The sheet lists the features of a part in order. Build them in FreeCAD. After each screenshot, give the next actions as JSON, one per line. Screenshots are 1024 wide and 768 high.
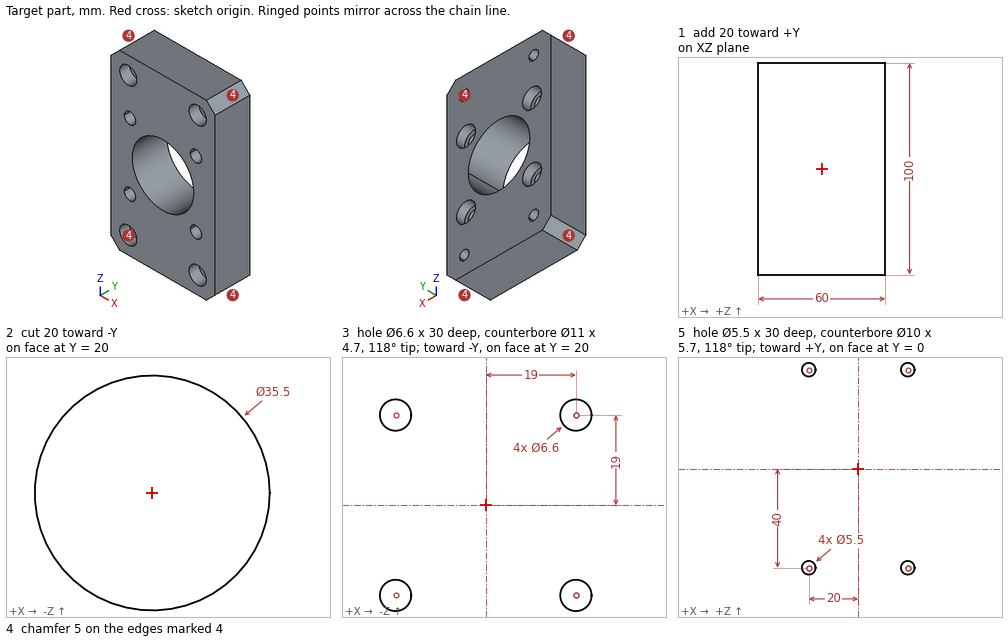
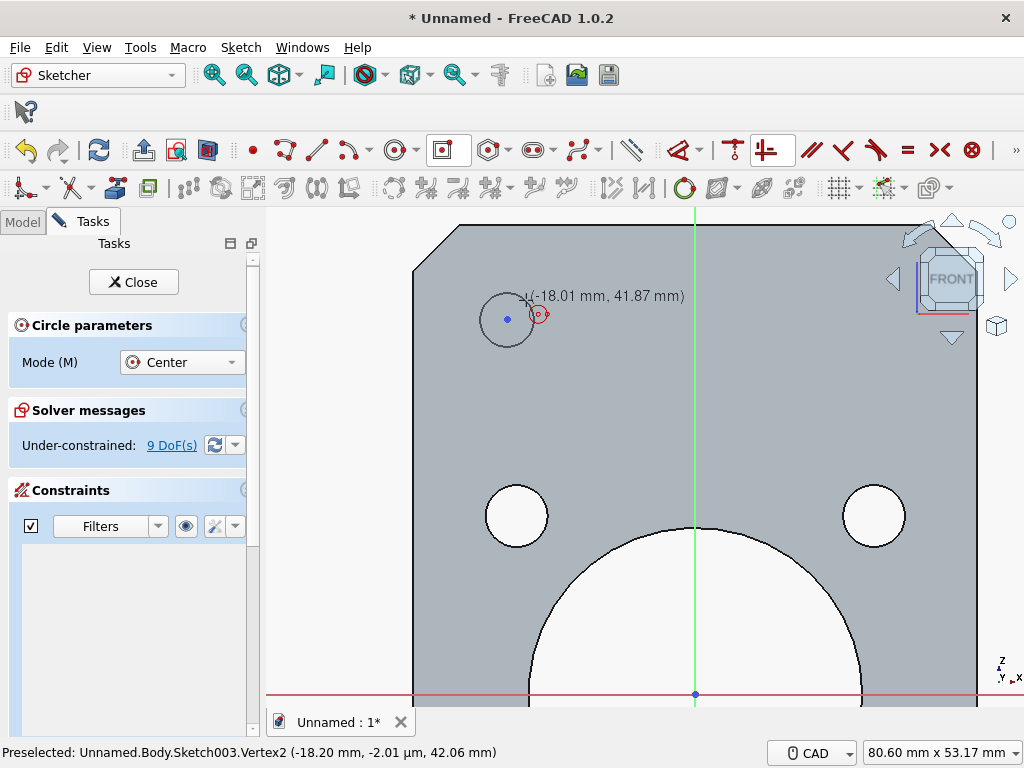
{"action": "scroll", "coordinate": [507, 319], "scroll_direction": "down", "scroll_amount": 5}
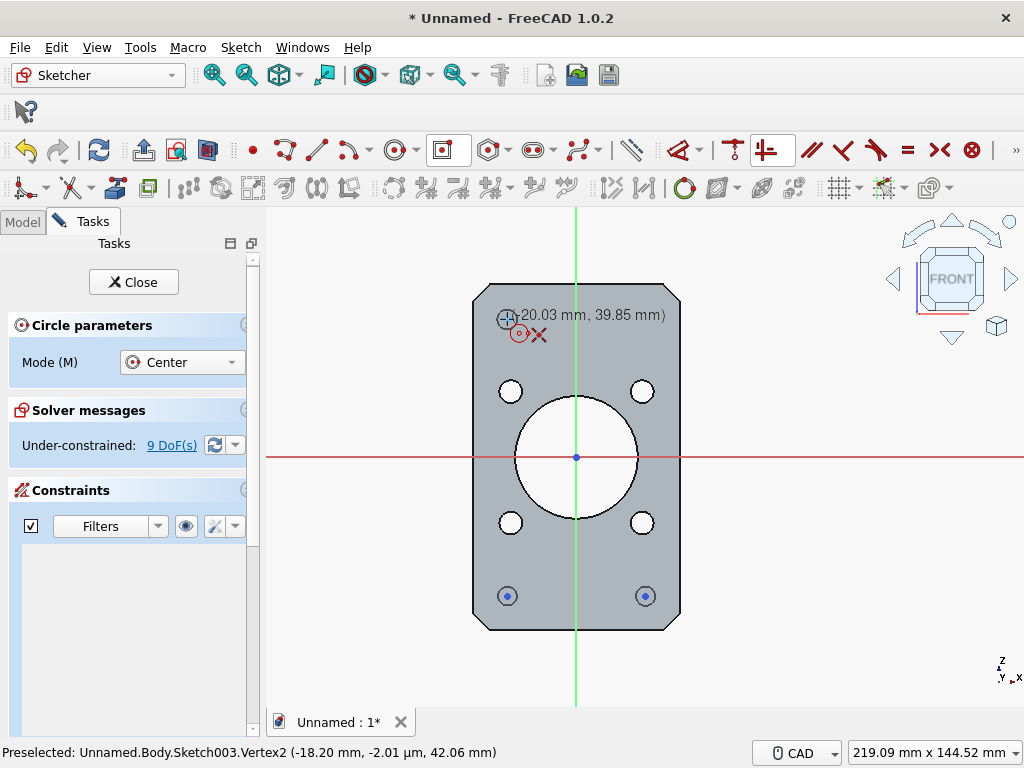
{"action": "scroll", "coordinate": [646, 319], "scroll_direction": "up", "scroll_amount": 5}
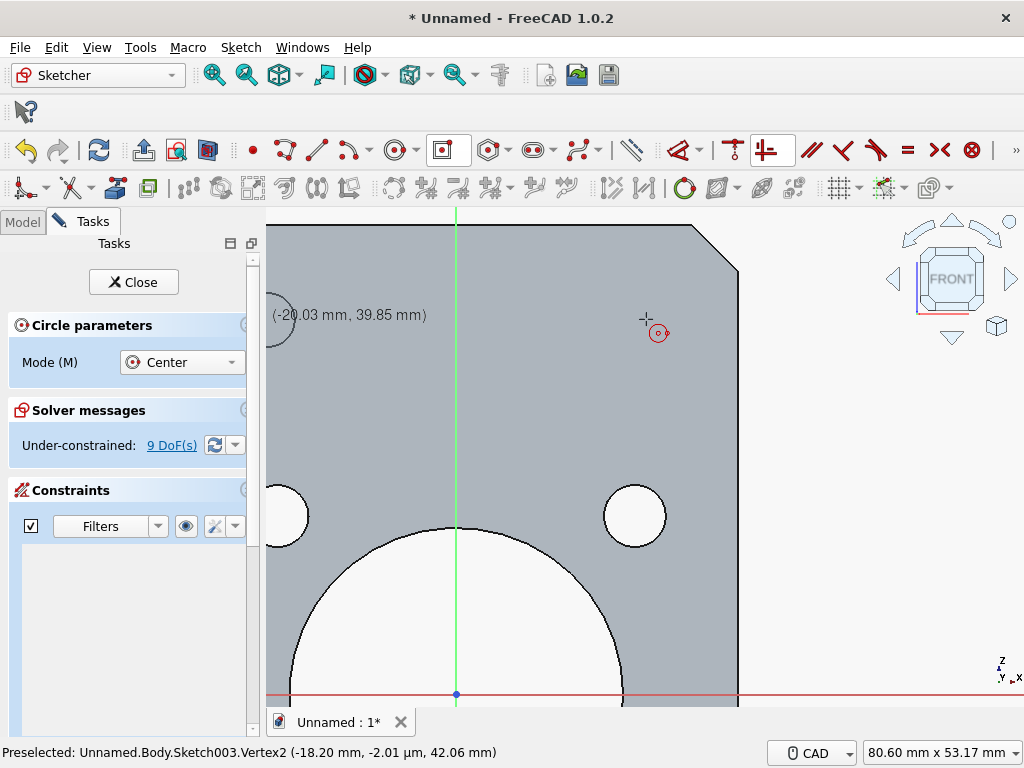
{"action": "left_click", "coordinate": [644, 319]}
{"action": "left_click", "coordinate": [663, 300]}
{"action": "key", "text": "Escape"}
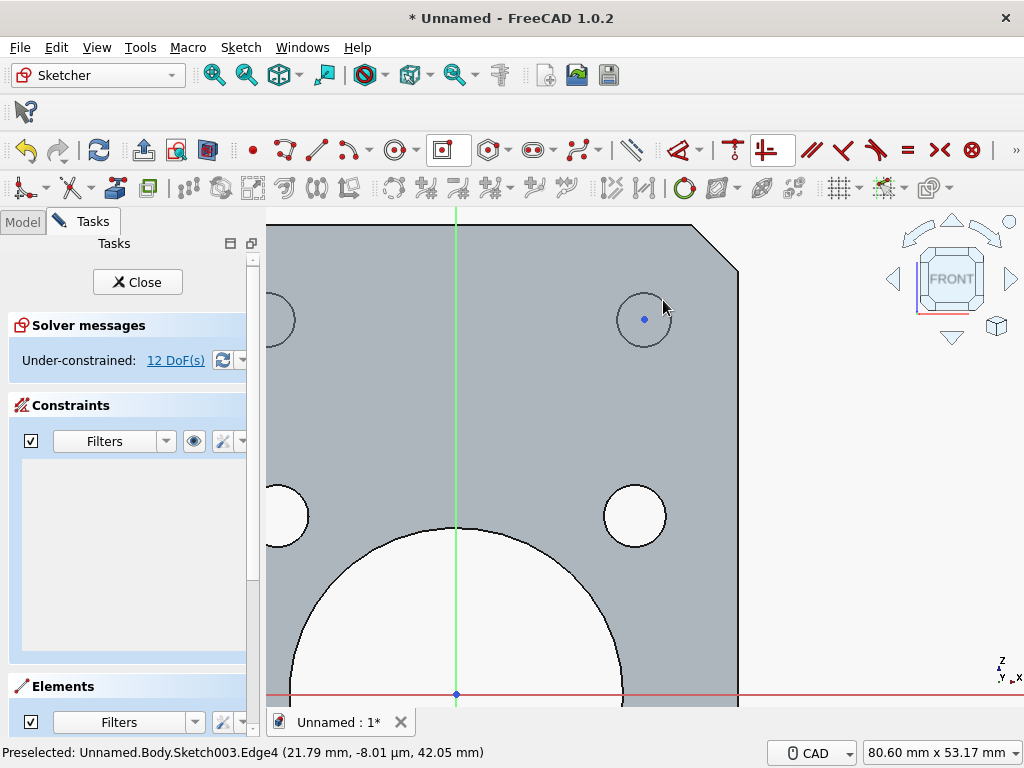
{"action": "scroll", "coordinate": [647, 319], "scroll_direction": "down", "scroll_amount": 5}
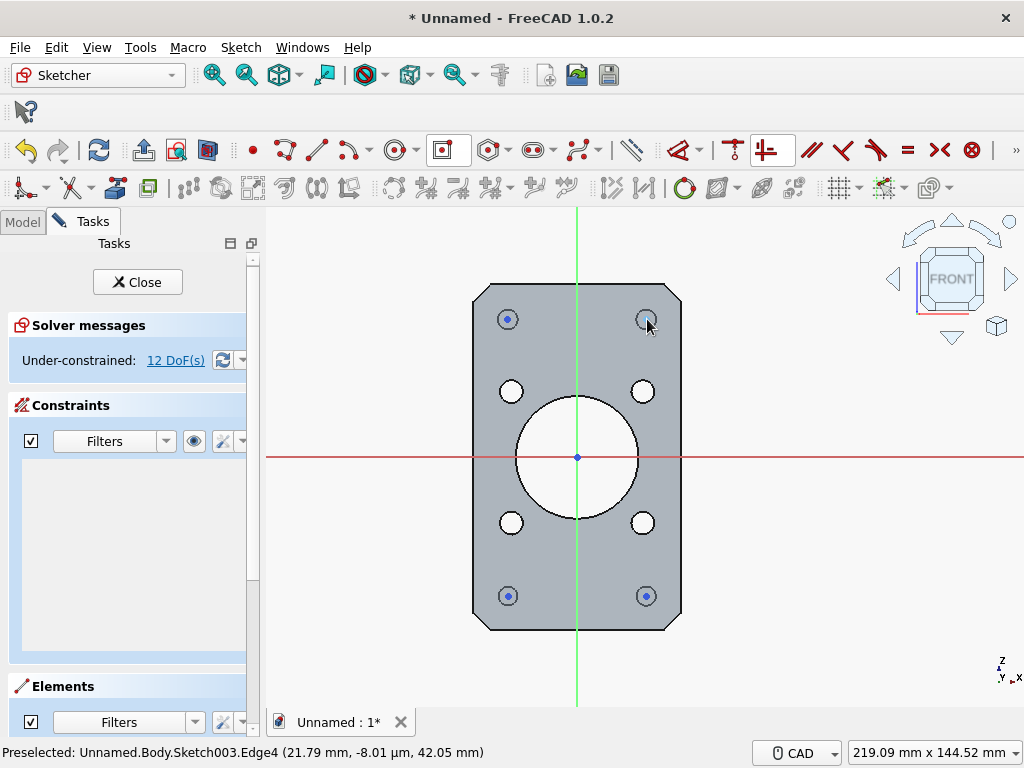
{"action": "scroll", "coordinate": [515, 589], "scroll_direction": "up", "scroll_amount": 2}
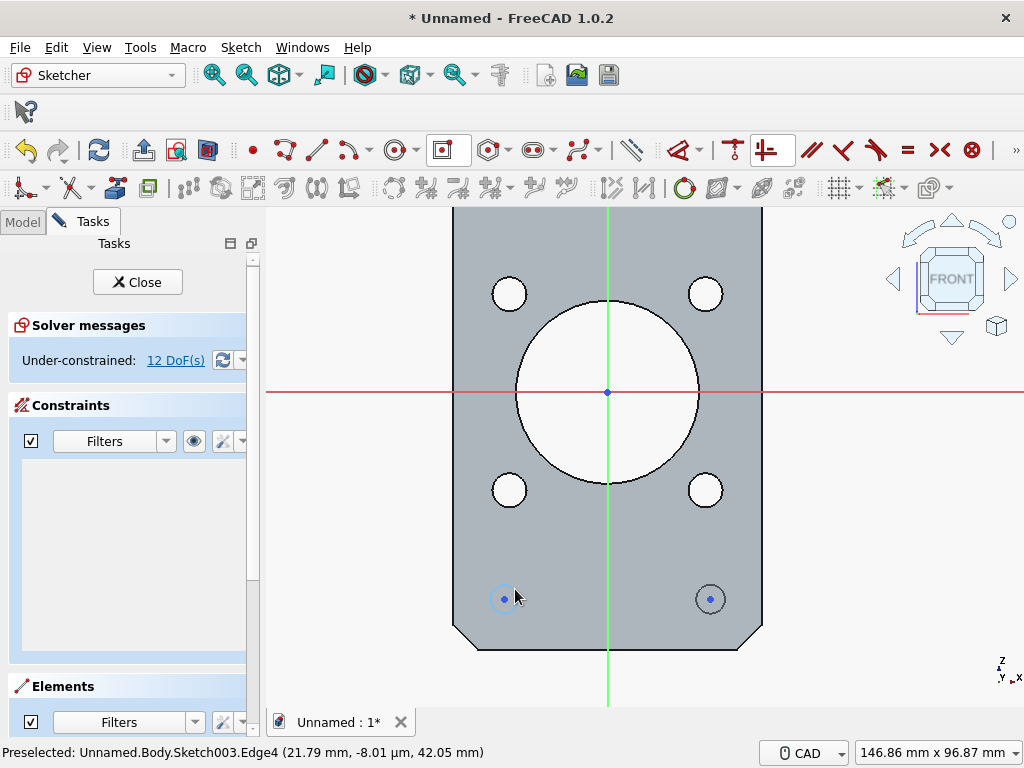
{"action": "left_click", "coordinate": [514, 589]}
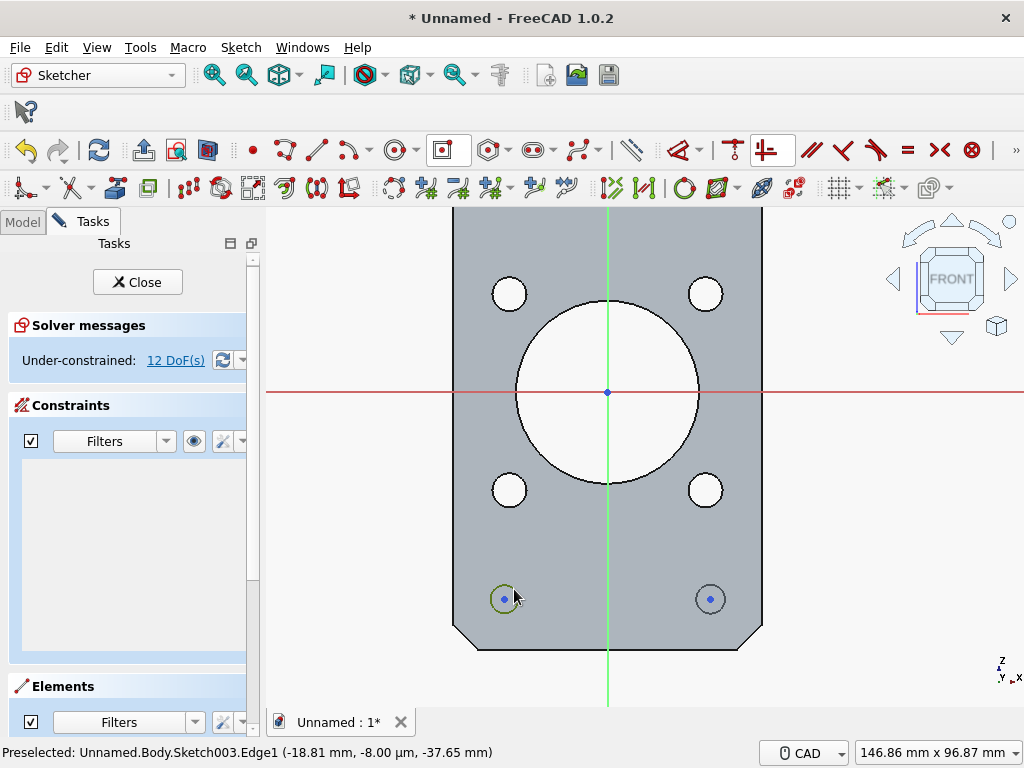
{"action": "left_click", "coordinate": [721, 589]}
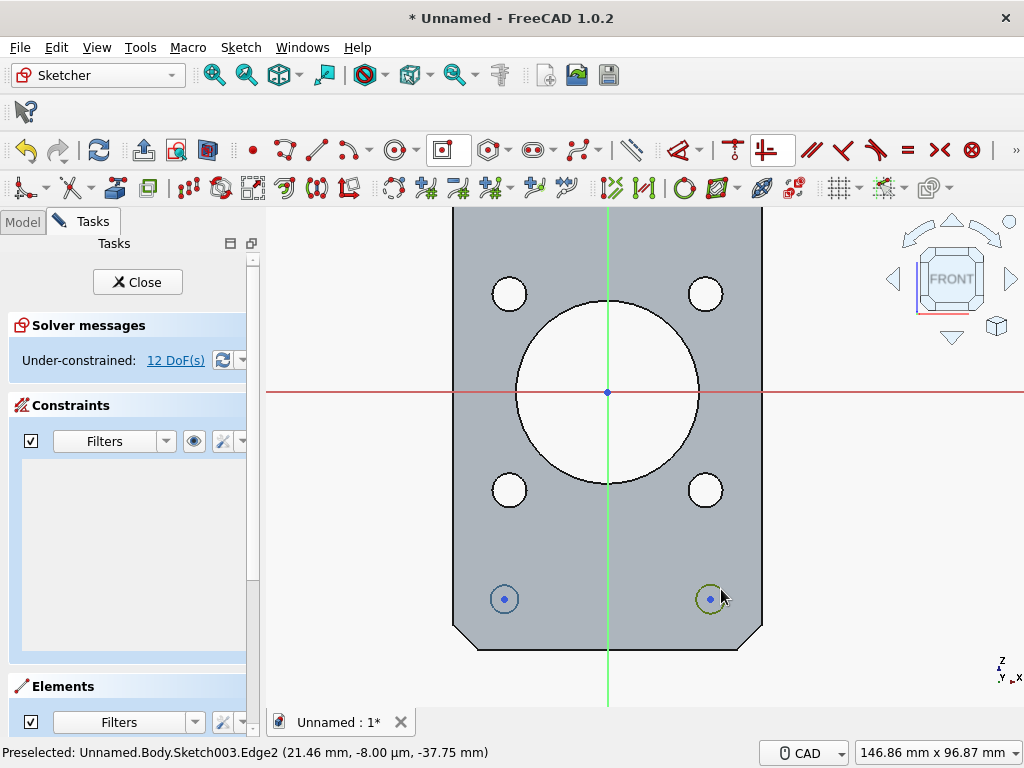
{"action": "scroll", "coordinate": [513, 589], "scroll_direction": "down", "scroll_amount": 2}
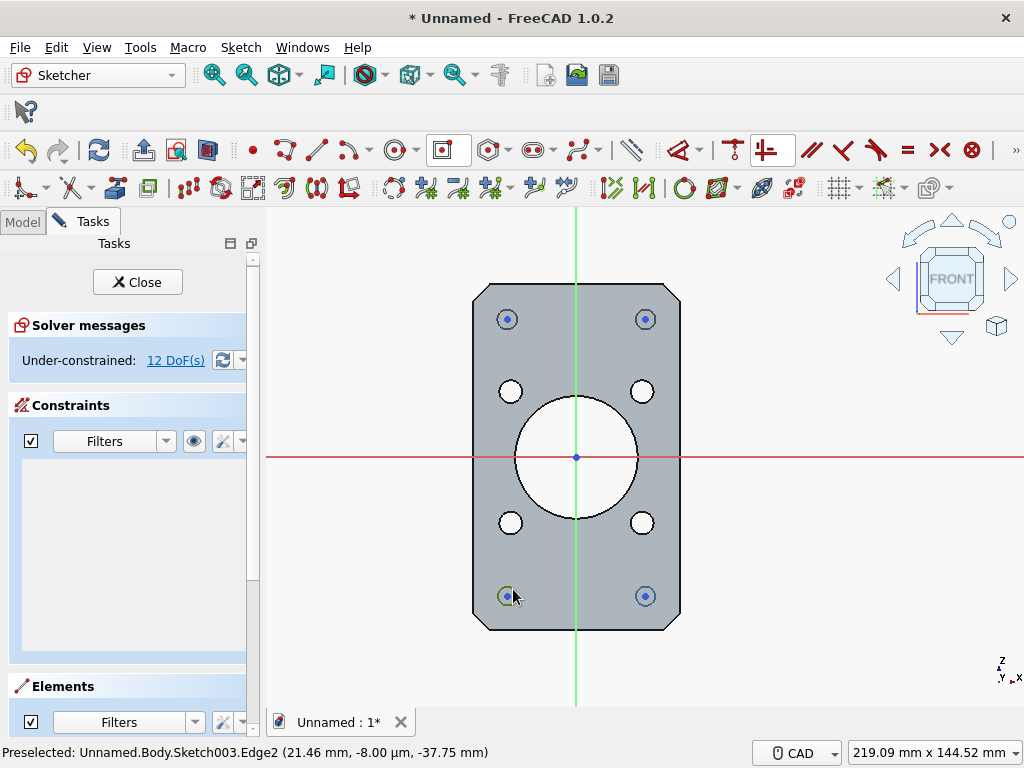
{"action": "scroll", "coordinate": [514, 312], "scroll_direction": "up", "scroll_amount": 2}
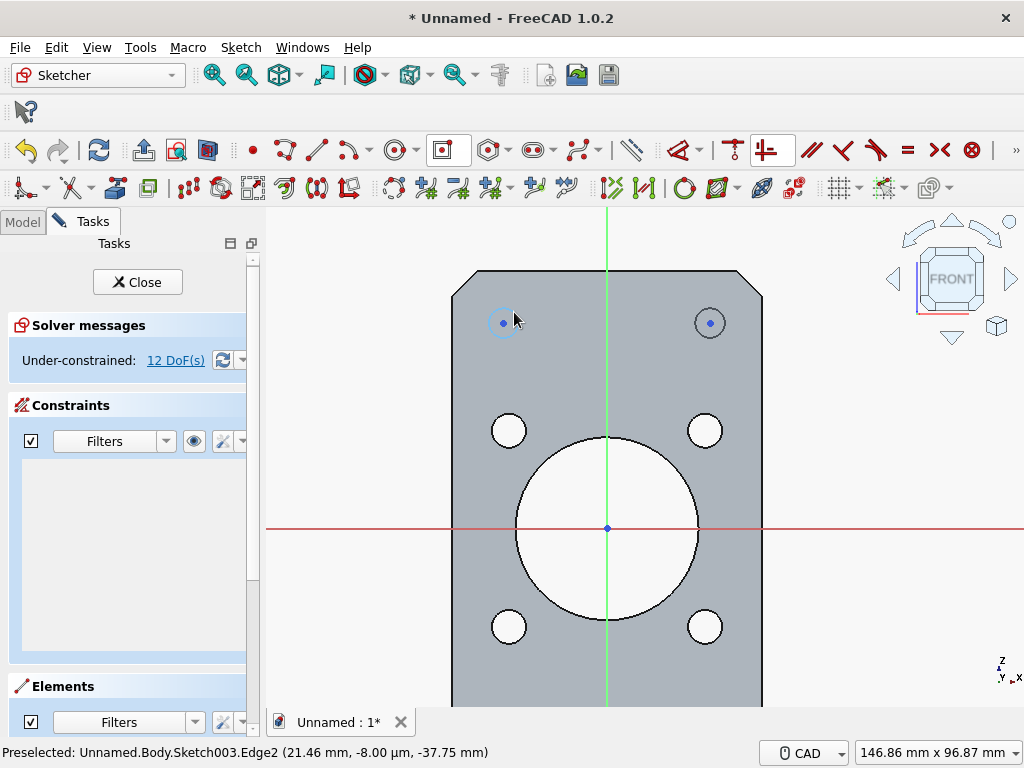
{"action": "left_click", "coordinate": [514, 313]}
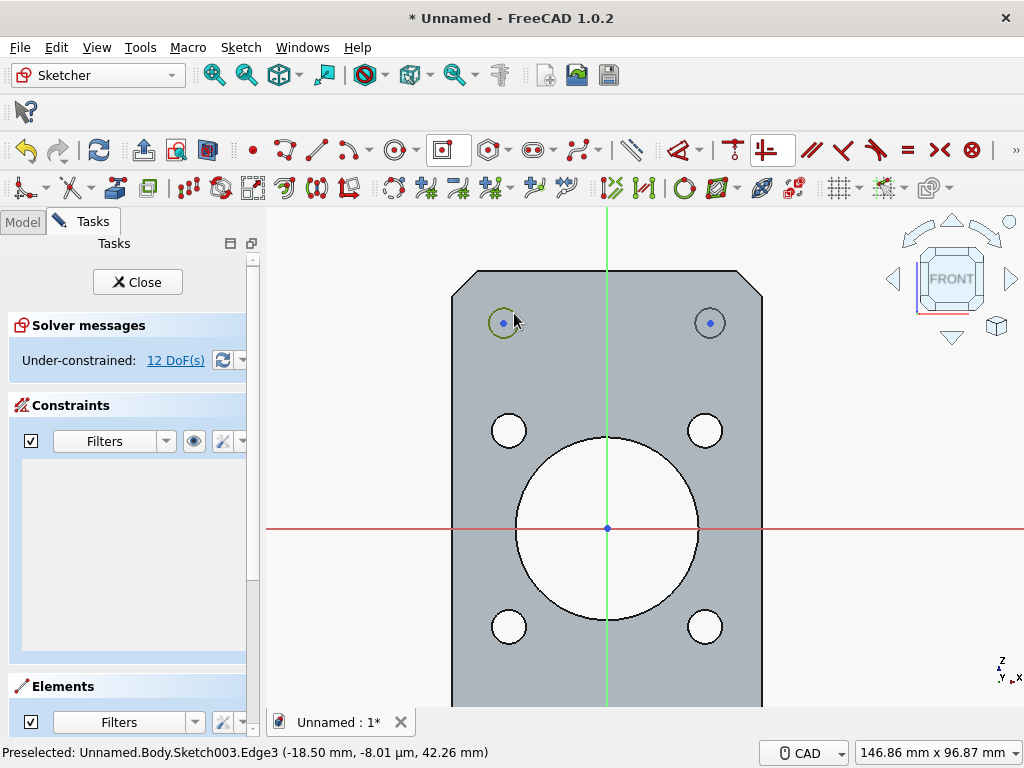
{"action": "left_click", "coordinate": [720, 313]}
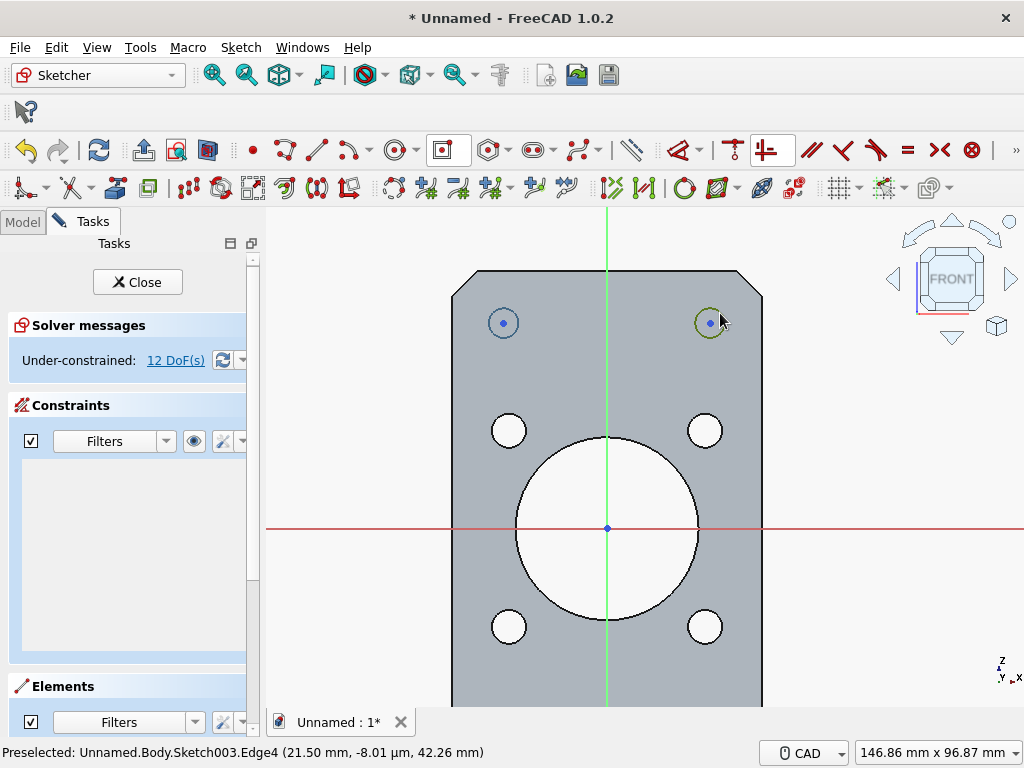
{"action": "key", "text": "e"}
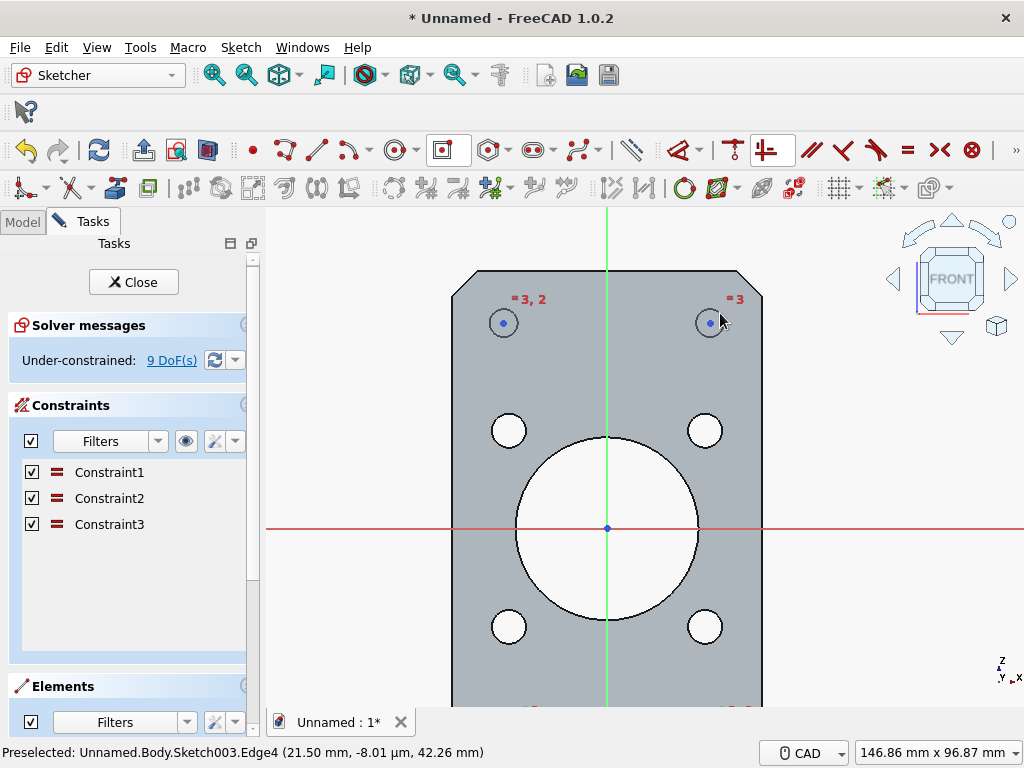
{"action": "scroll", "coordinate": [514, 311], "scroll_direction": "down", "scroll_amount": 2}